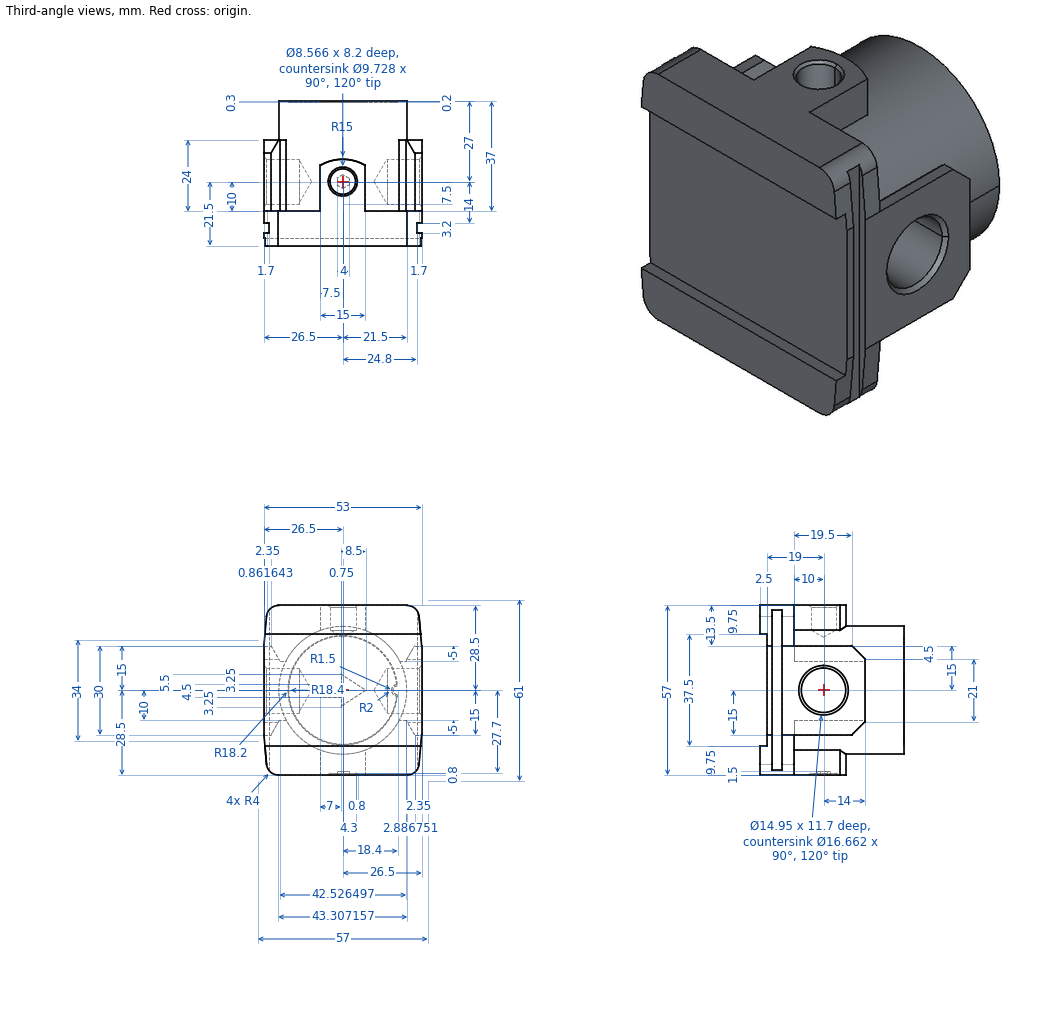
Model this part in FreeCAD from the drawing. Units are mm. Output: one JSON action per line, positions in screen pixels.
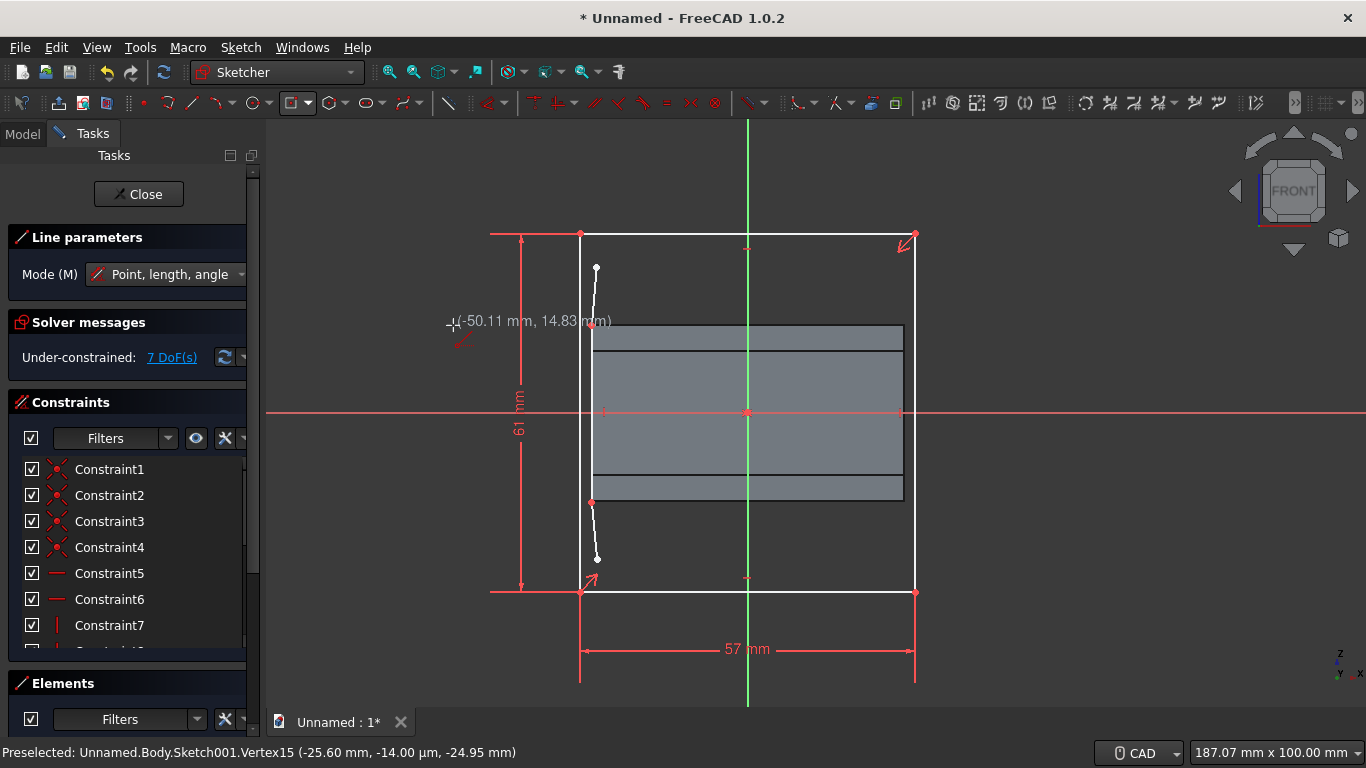
{"action": "scroll", "coordinate": [620, 581], "scroll_direction": "up", "scroll_amount": 2}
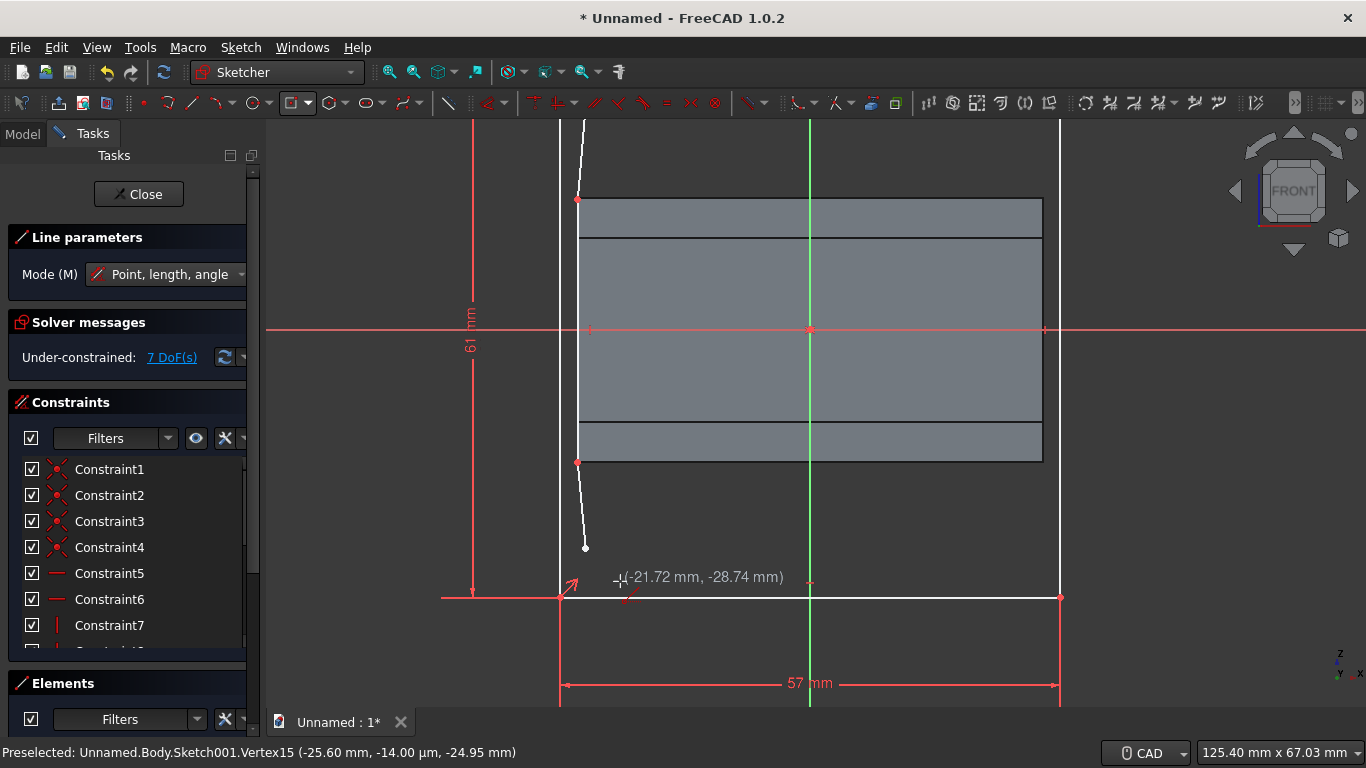
{"action": "left_click", "coordinate": [620, 580]}
{"action": "left_click", "coordinate": [1000, 580]}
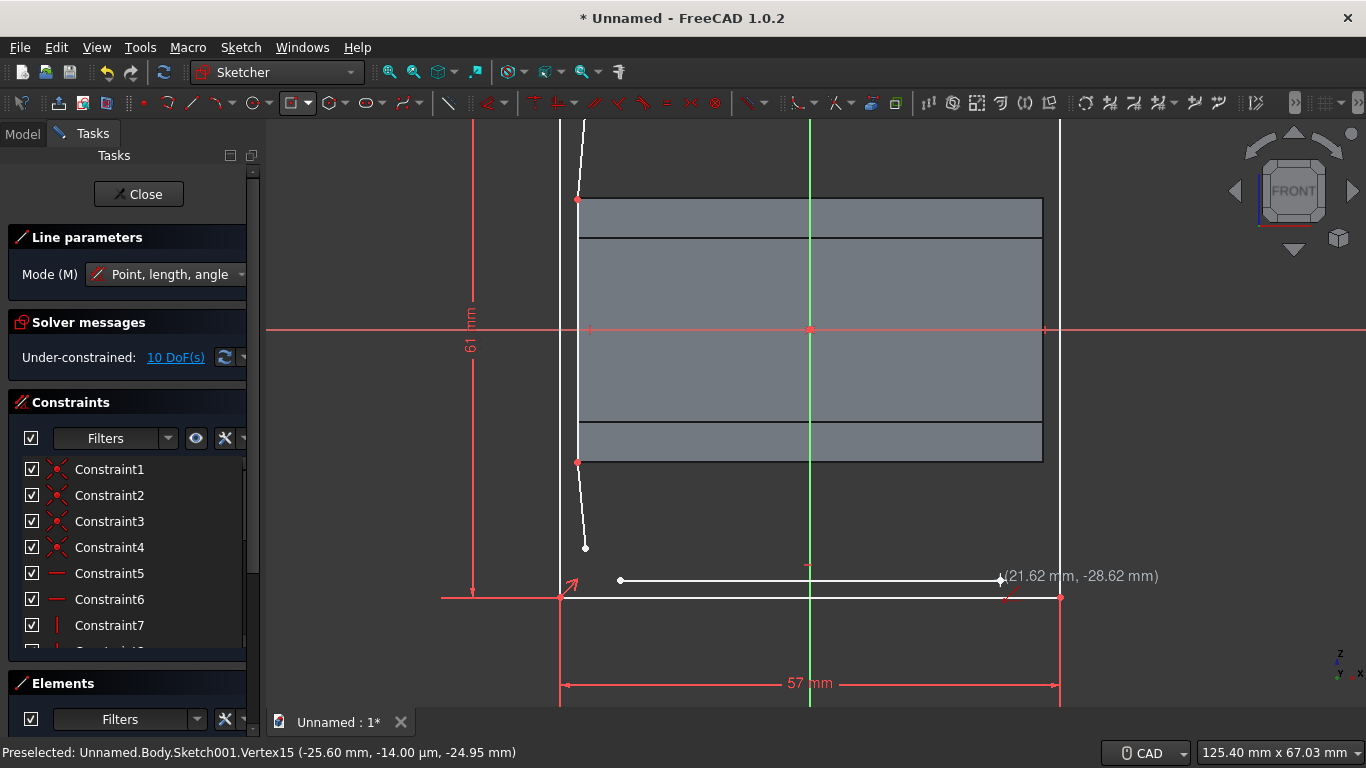
{"action": "left_click", "coordinate": [168, 104]}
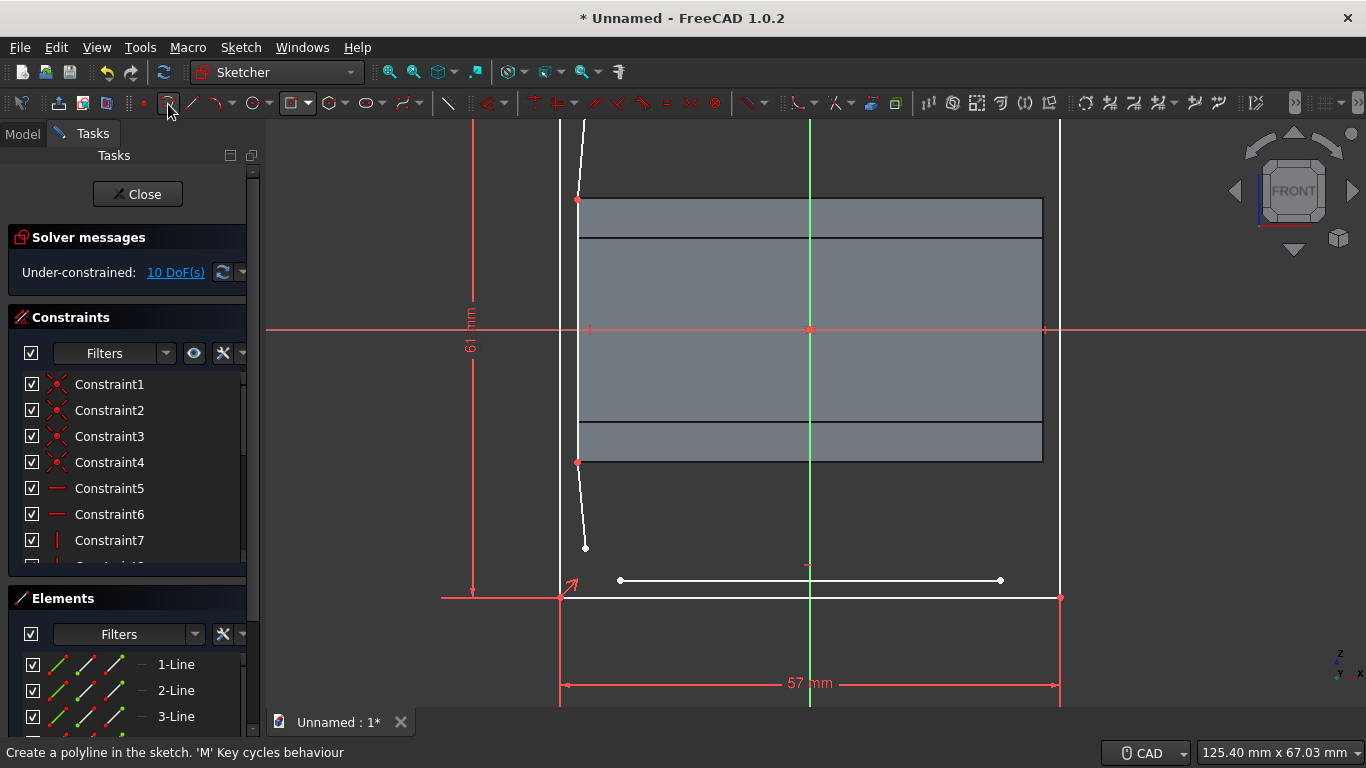
{"action": "left_click", "coordinate": [1035, 548]}
{"action": "left_click", "coordinate": [1043, 462]}
{"action": "left_click", "coordinate": [1043, 198]}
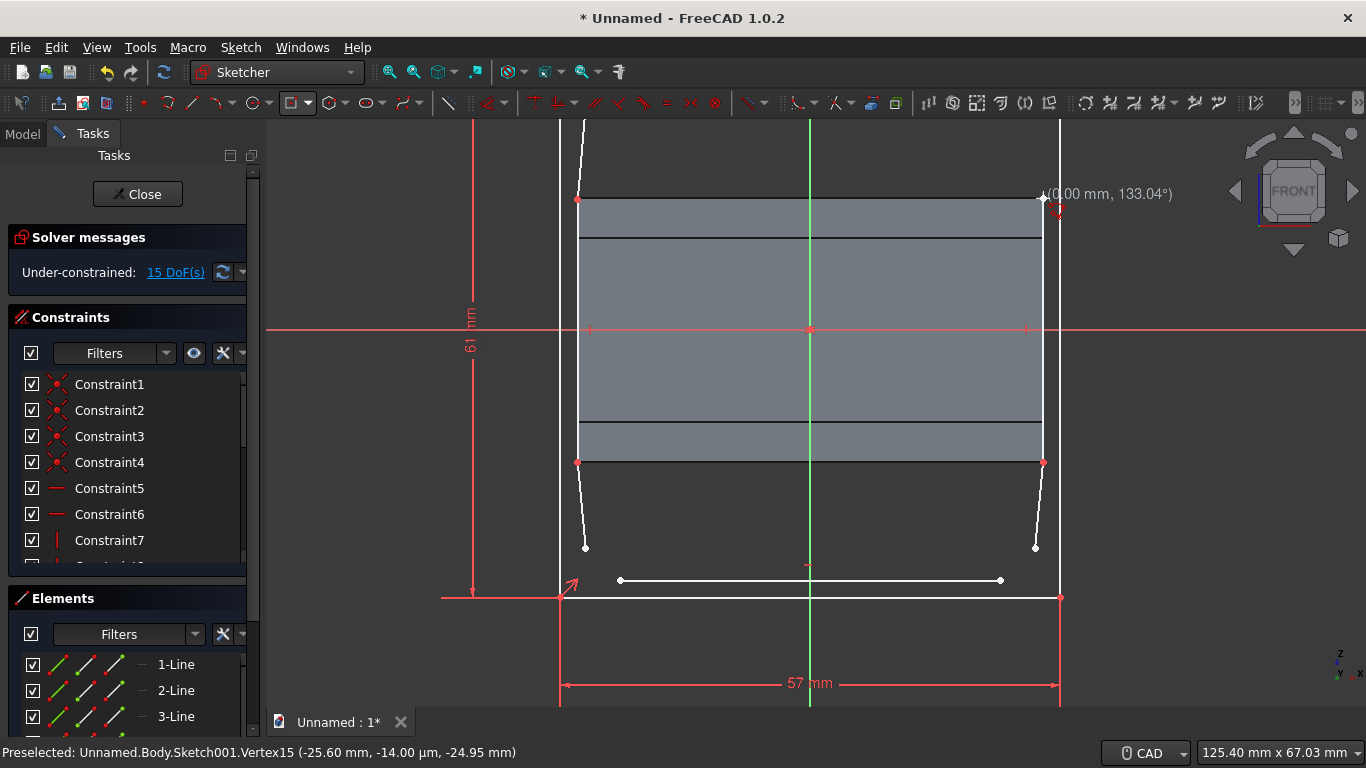
{"action": "scroll", "coordinate": [620, 582], "scroll_direction": "down", "scroll_amount": 2}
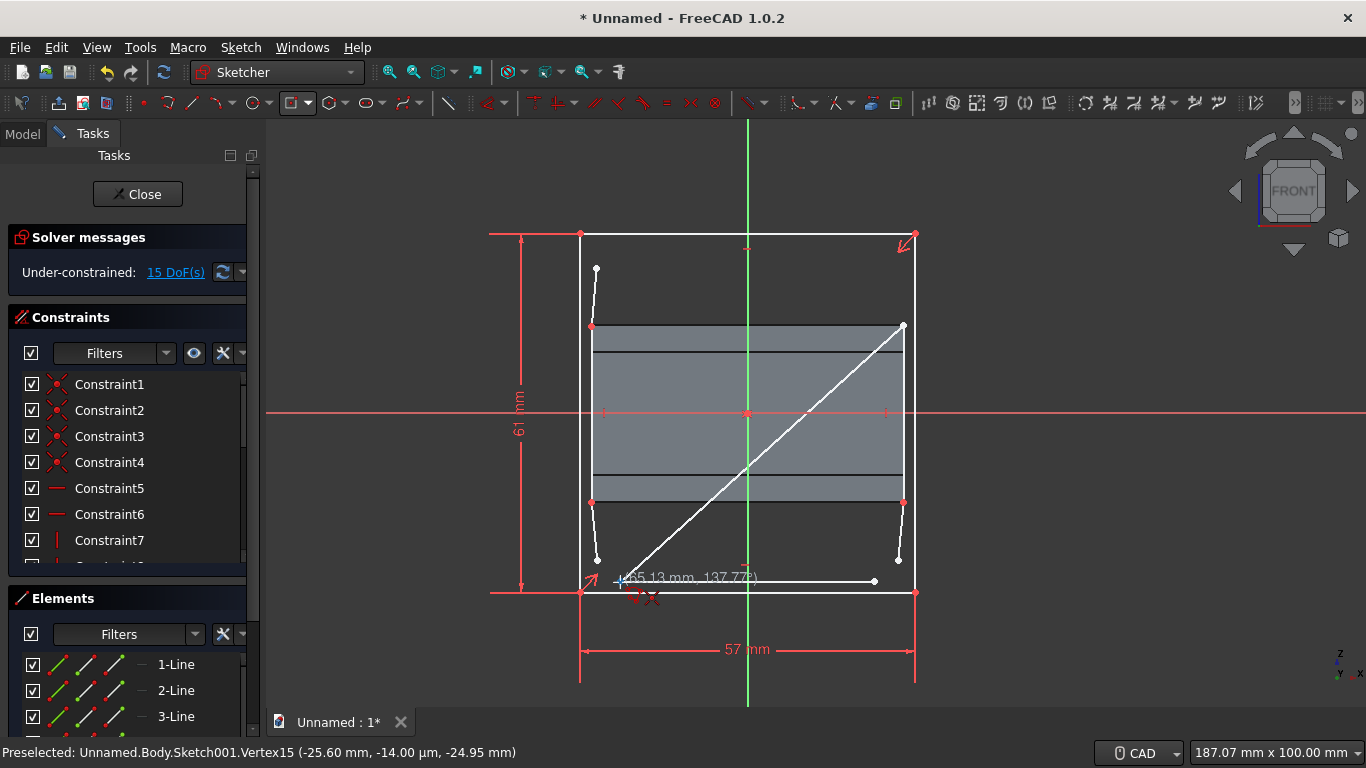
{"action": "left_click", "coordinate": [898, 267]}
{"action": "right_click", "coordinate": [898, 267]}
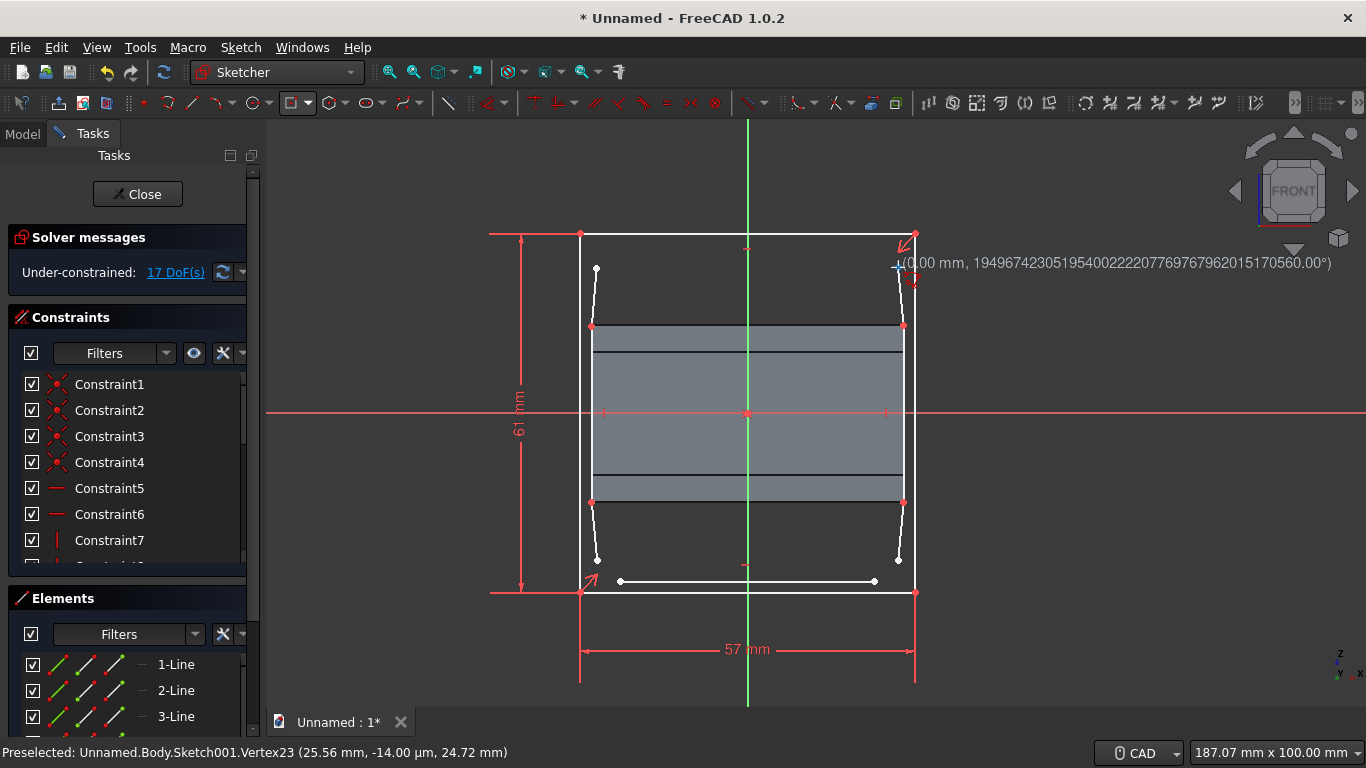
{"action": "key", "text": "g l"}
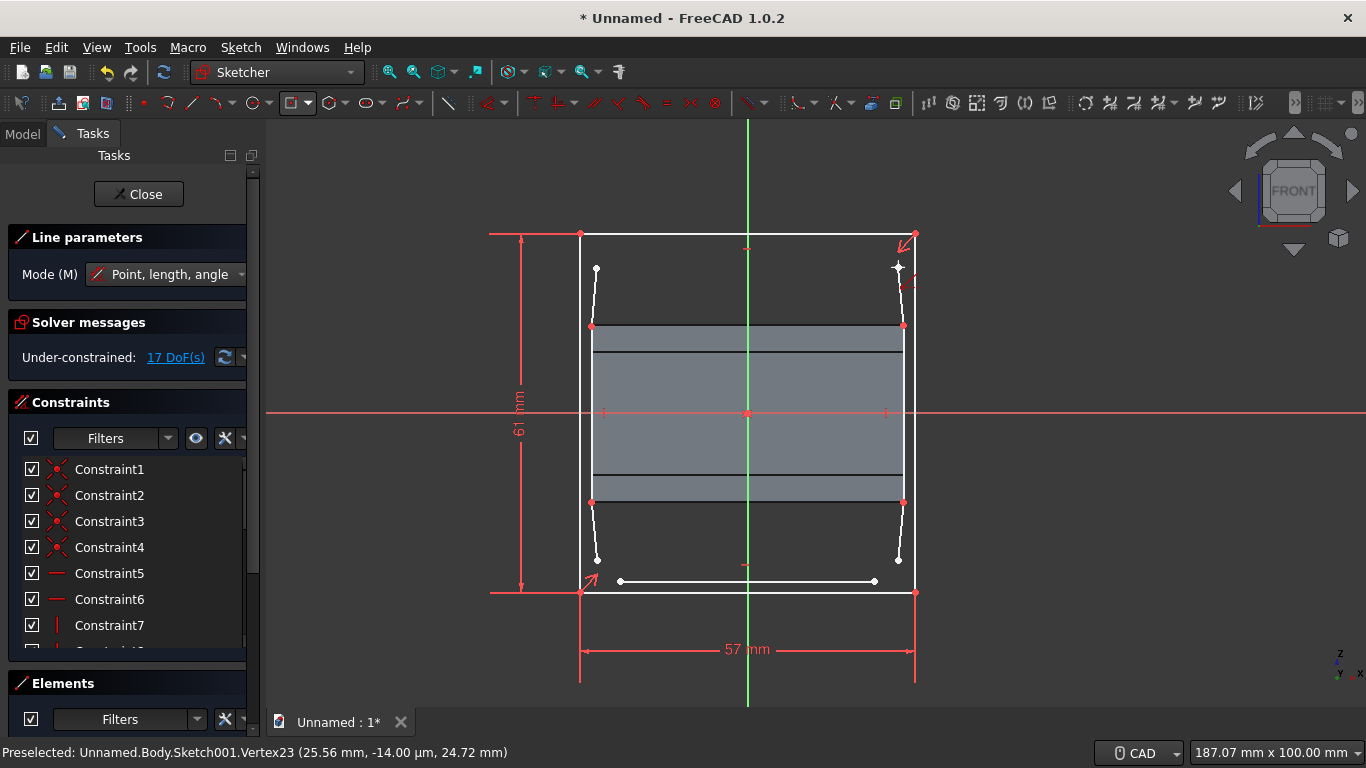
{"action": "scroll", "coordinate": [875, 246], "scroll_direction": "up", "scroll_amount": 2}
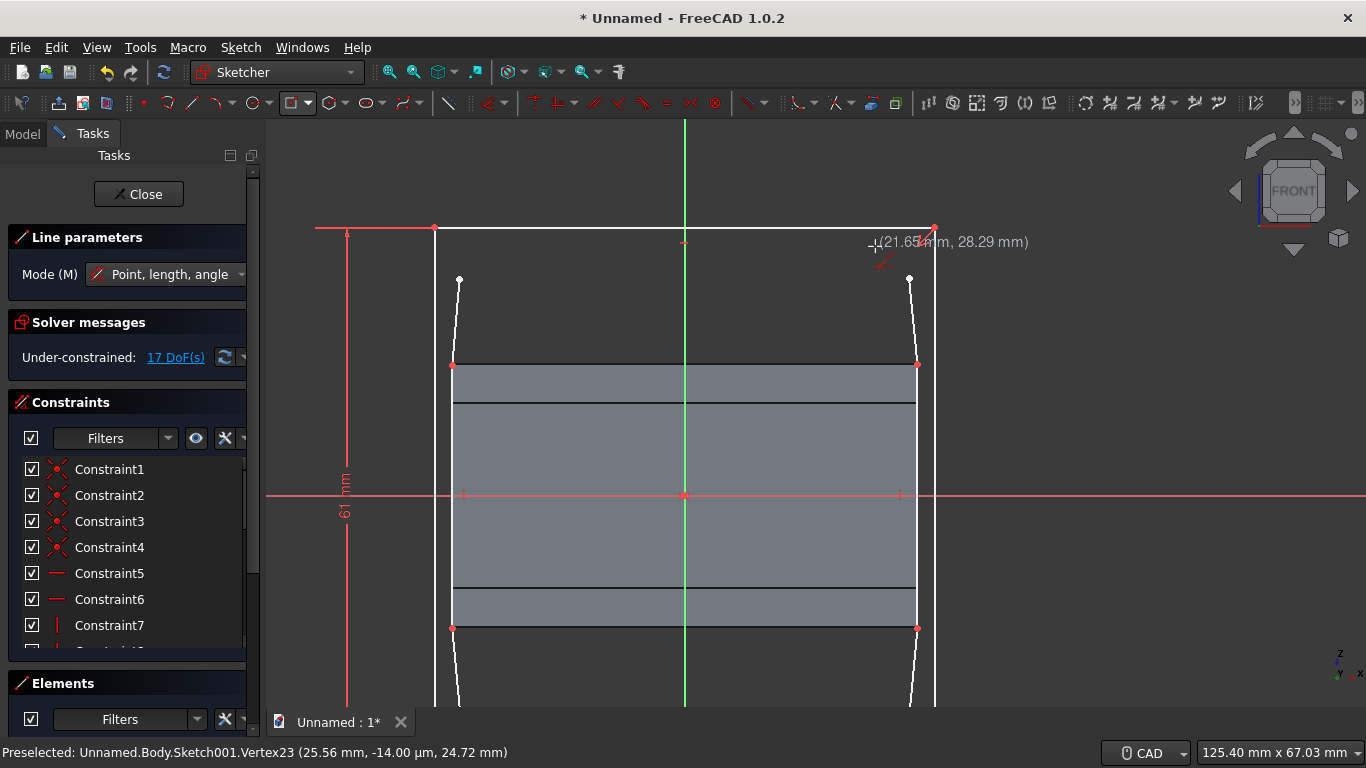
{"action": "left_click", "coordinate": [875, 246]}
{"action": "left_click", "coordinate": [495, 246]}